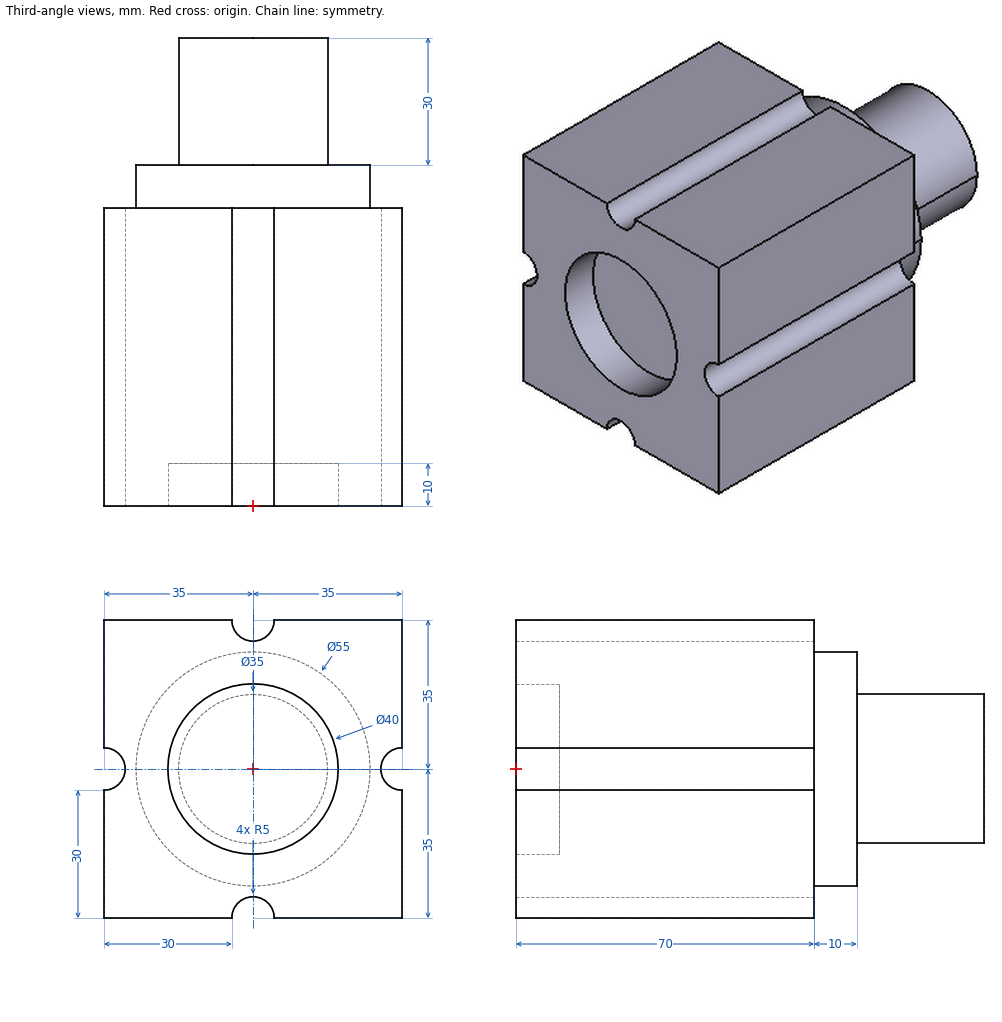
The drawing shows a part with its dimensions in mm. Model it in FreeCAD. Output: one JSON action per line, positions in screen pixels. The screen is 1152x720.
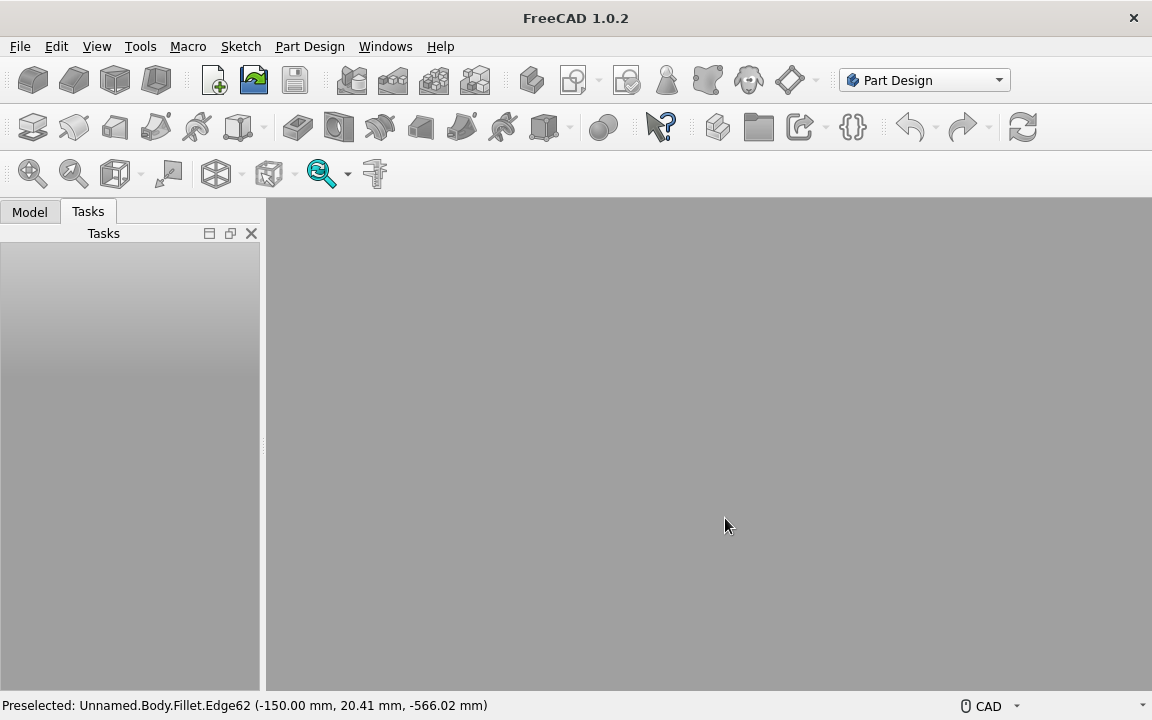
{"action": "left_click", "coordinate": [213, 80]}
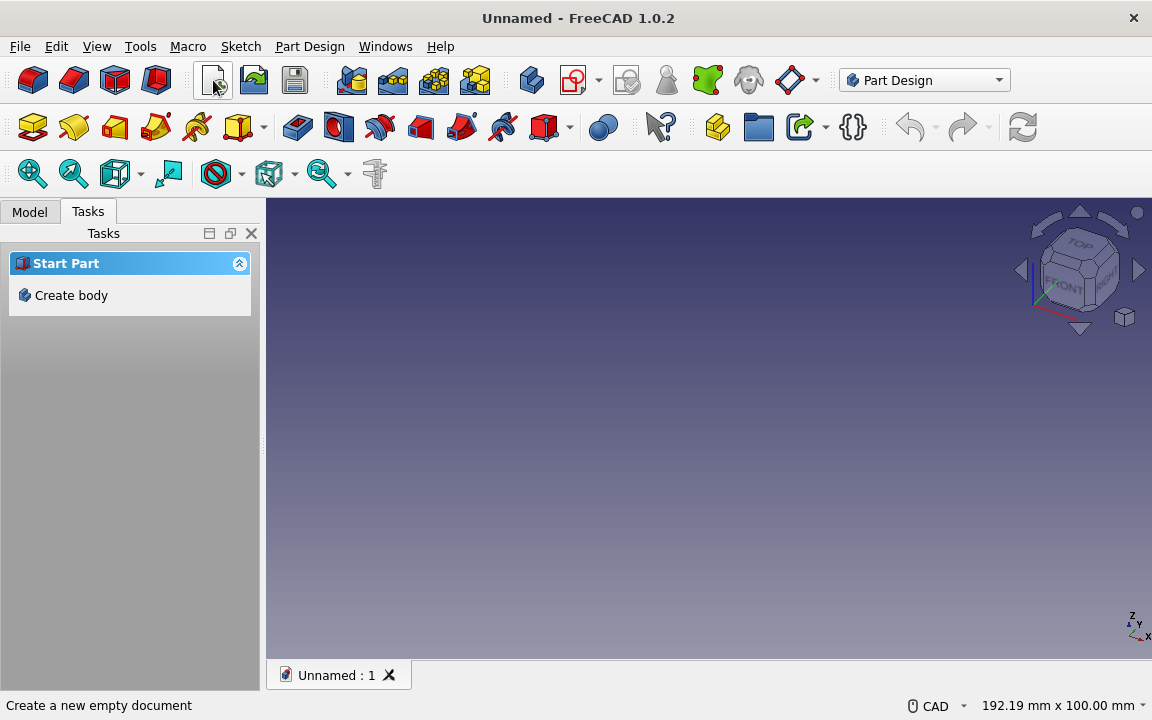
{"action": "left_click", "coordinate": [572, 80]}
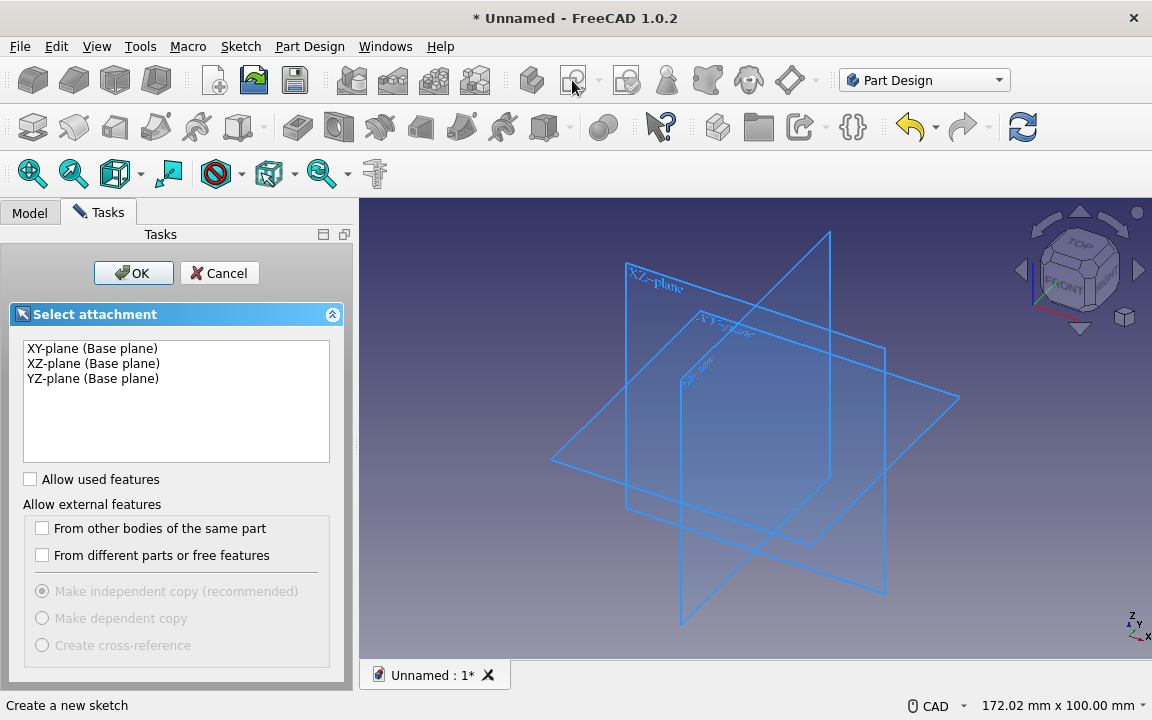
{"action": "left_click", "coordinate": [84, 364]}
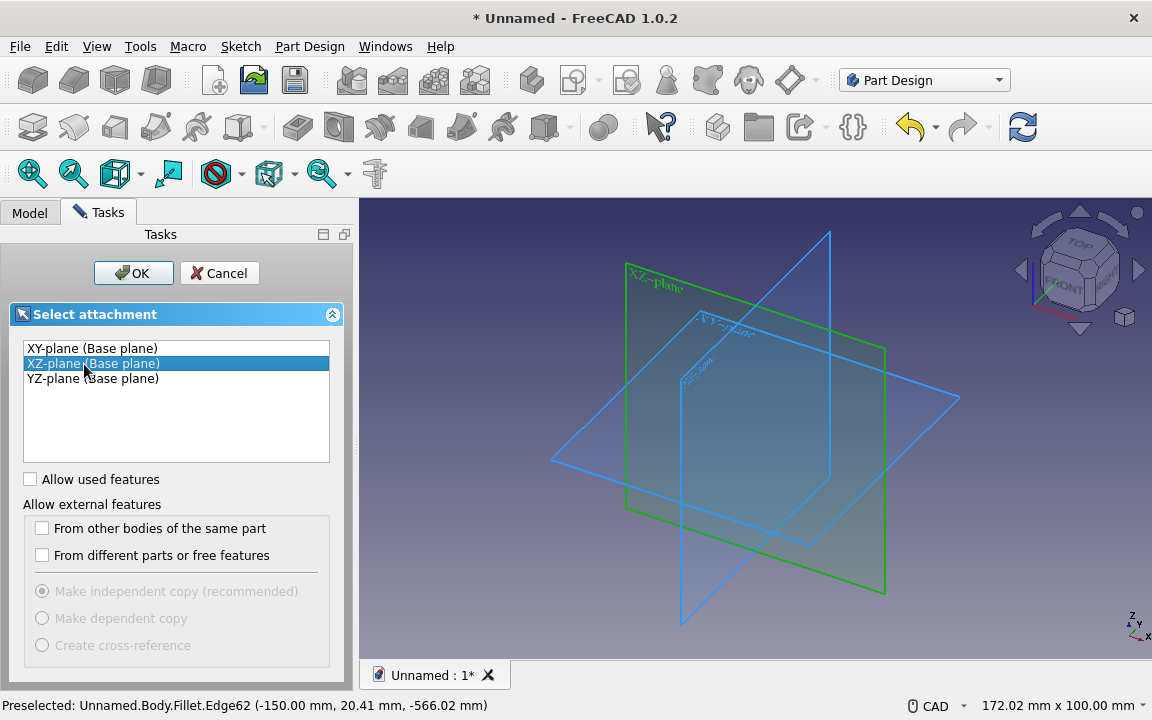
{"action": "left_click", "coordinate": [134, 273]}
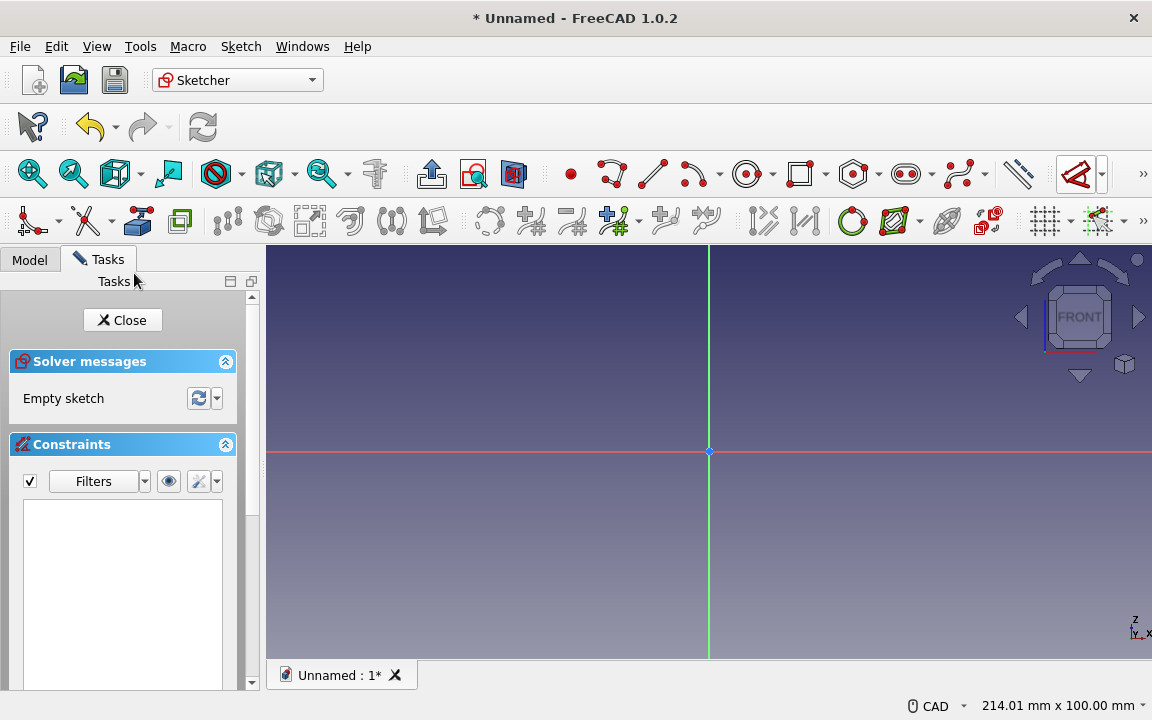
{"action": "left_click", "coordinate": [612, 174]}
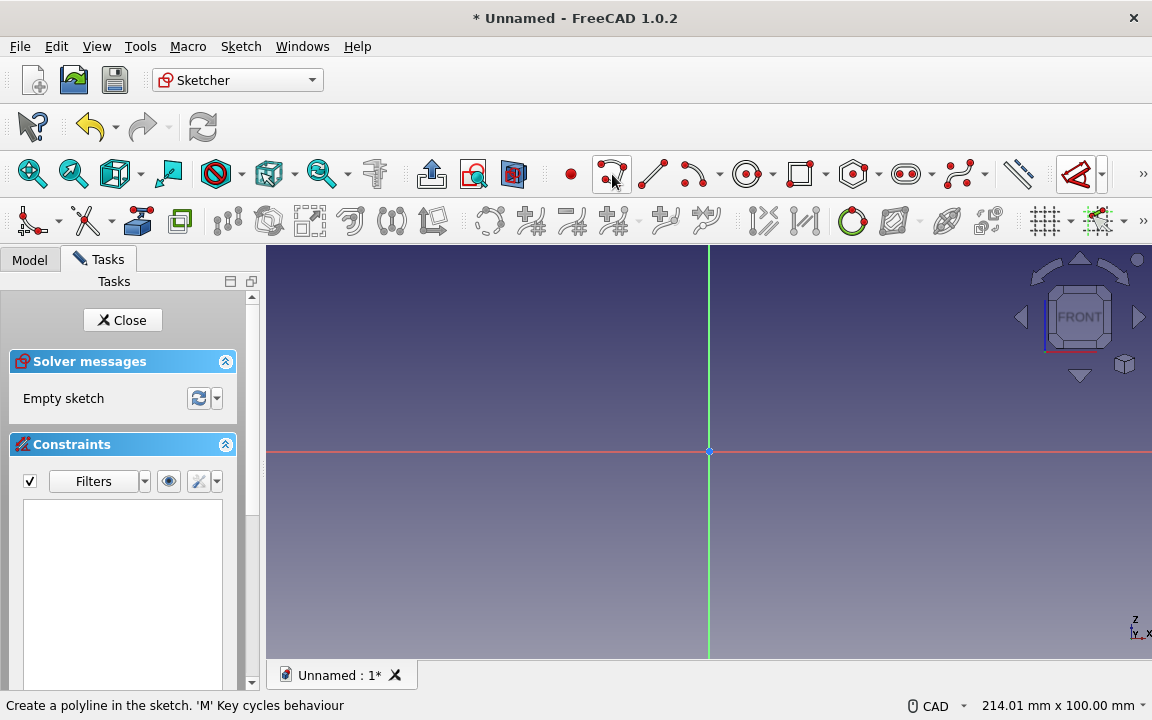
{"action": "left_click", "coordinate": [688, 597]}
{"action": "left_click", "coordinate": [564, 597]}
{"action": "left_click", "coordinate": [564, 473]}
{"action": "right_click", "coordinate": [564, 473]}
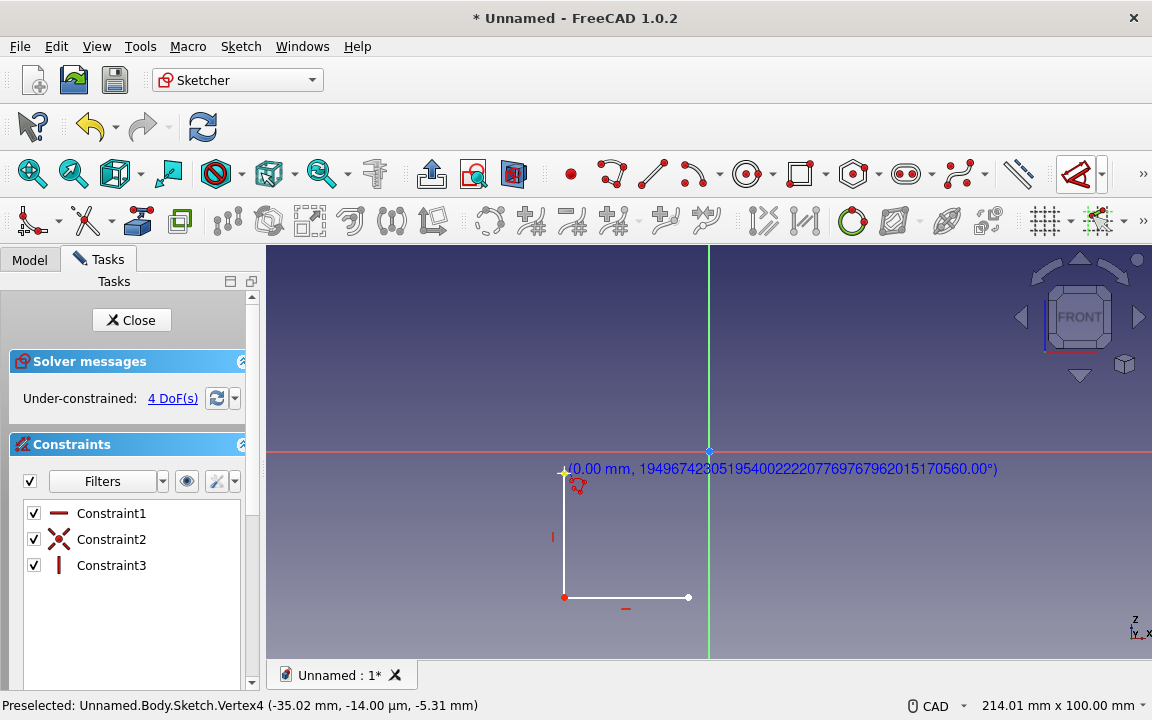
{"action": "left_click", "coordinate": [564, 431]}
{"action": "left_click", "coordinate": [564, 307]}
{"action": "left_click", "coordinate": [688, 307]}
{"action": "right_click", "coordinate": [688, 307]}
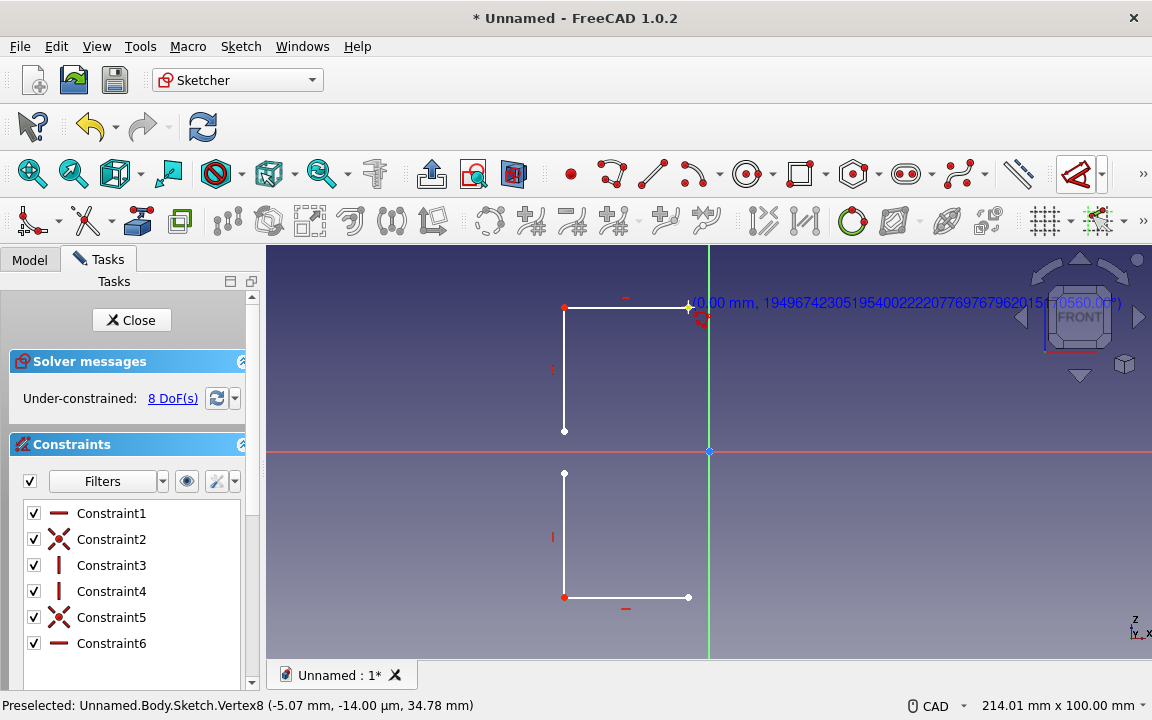
{"action": "left_click", "coordinate": [730, 307]}
{"action": "left_click", "coordinate": [854, 307]}
{"action": "left_click", "coordinate": [854, 431]}
{"action": "right_click", "coordinate": [854, 431]}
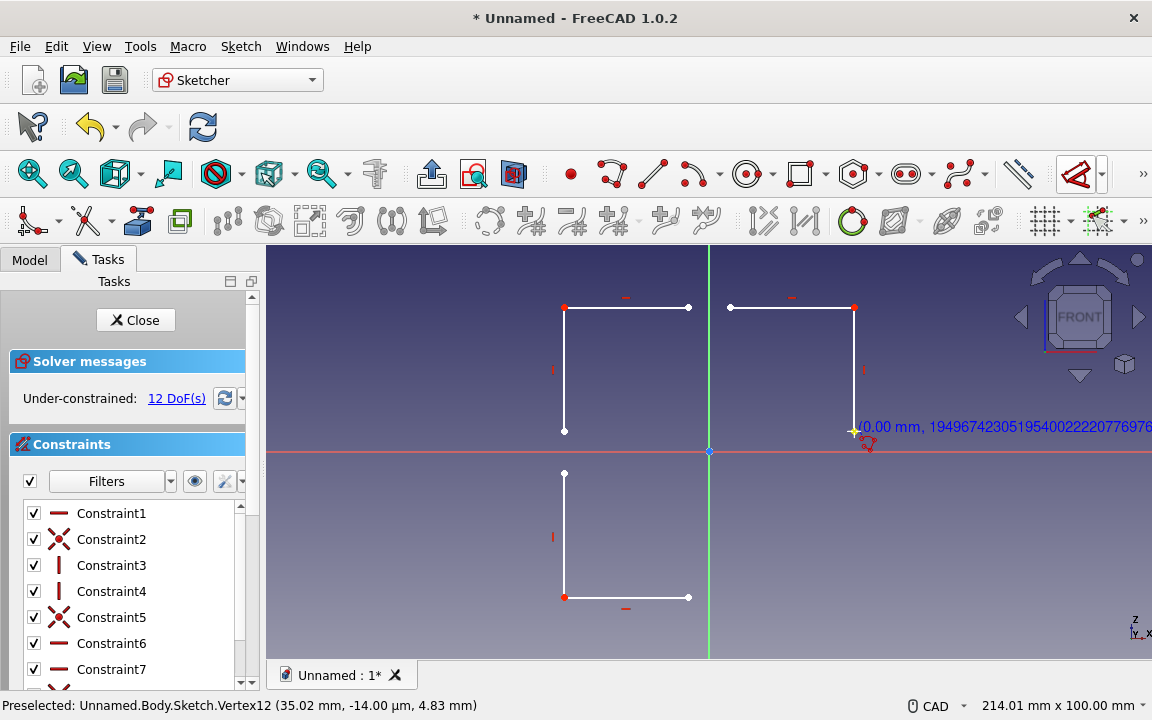
{"action": "left_click", "coordinate": [854, 473]}
{"action": "left_click", "coordinate": [854, 597]}
{"action": "left_click", "coordinate": [730, 597]}
{"action": "right_click", "coordinate": [730, 597]}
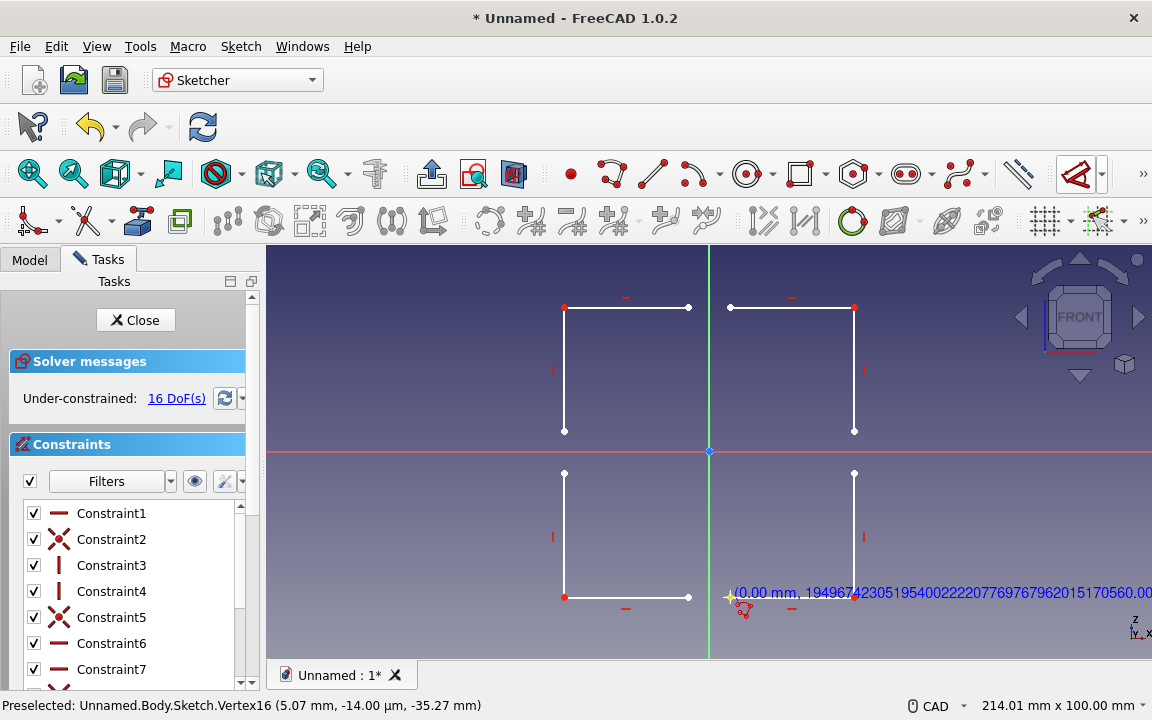
{"action": "key", "text": "g 3 a"}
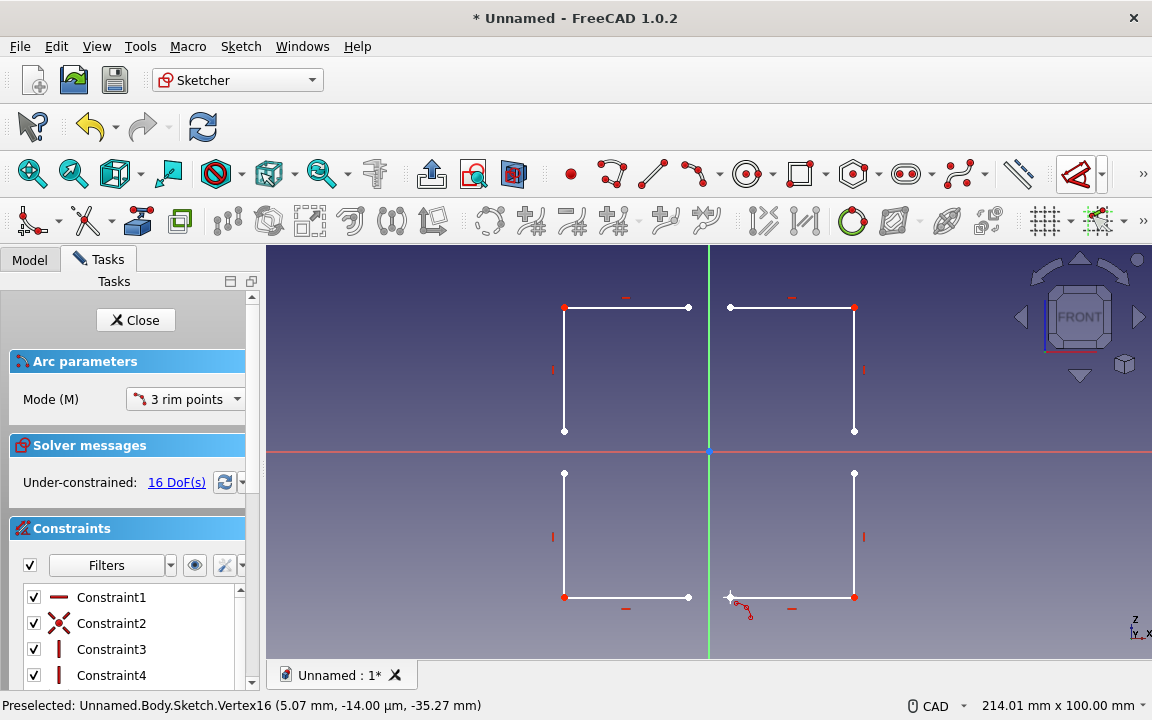
{"action": "left_click", "coordinate": [564, 474]}
{"action": "left_click", "coordinate": [564, 432]}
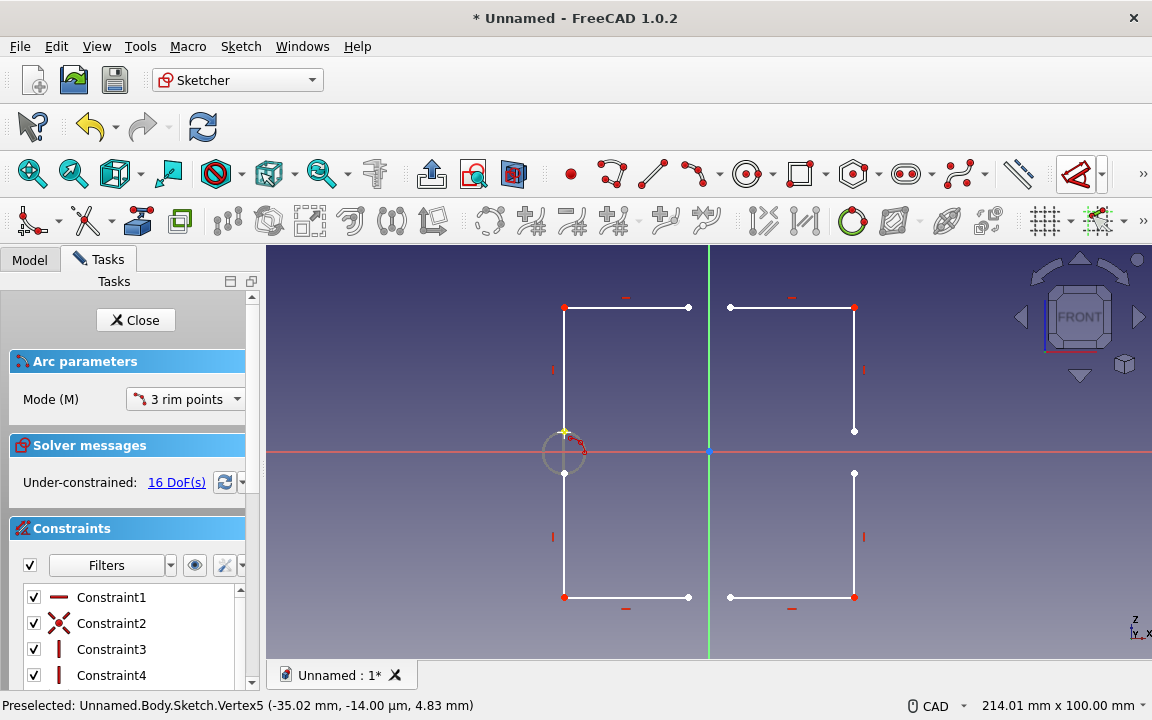
{"action": "scroll", "coordinate": [581, 464], "scroll_direction": "up", "scroll_amount": 2}